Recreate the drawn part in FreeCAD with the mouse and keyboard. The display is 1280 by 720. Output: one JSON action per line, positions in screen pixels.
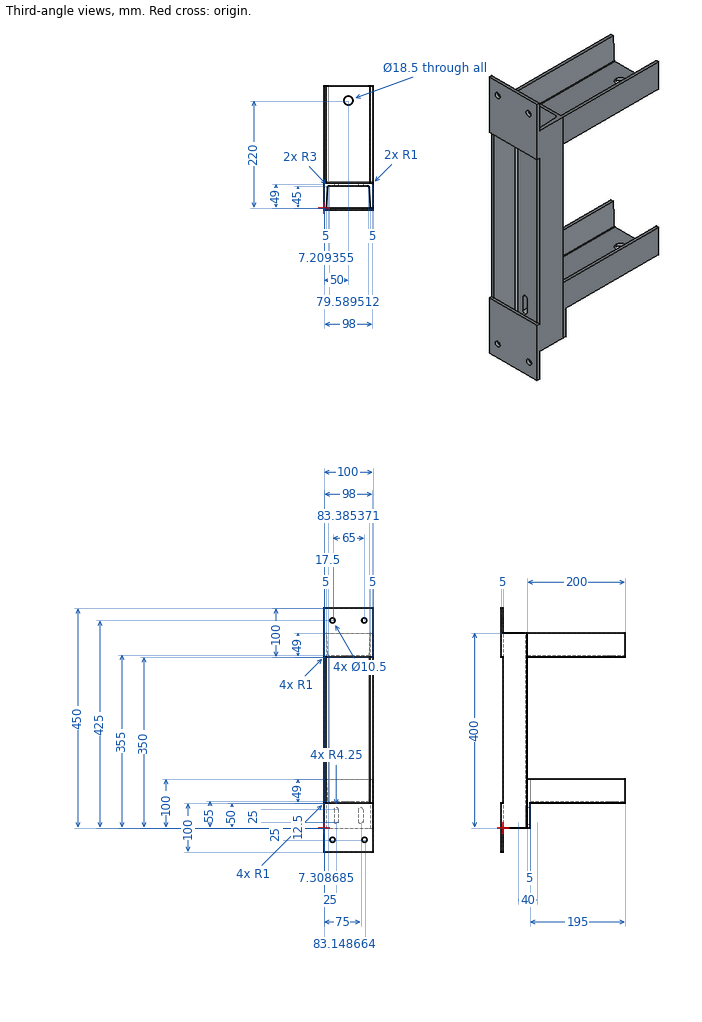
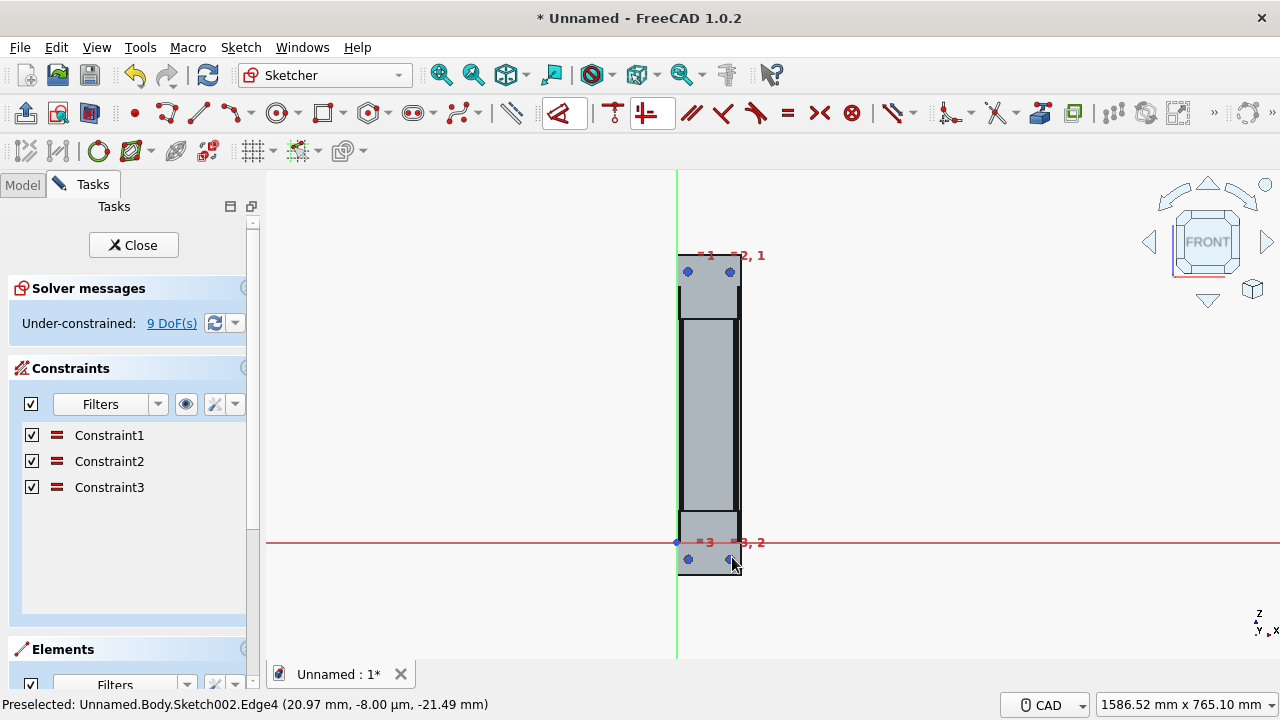
{"action": "left_click", "coordinate": [688, 272]}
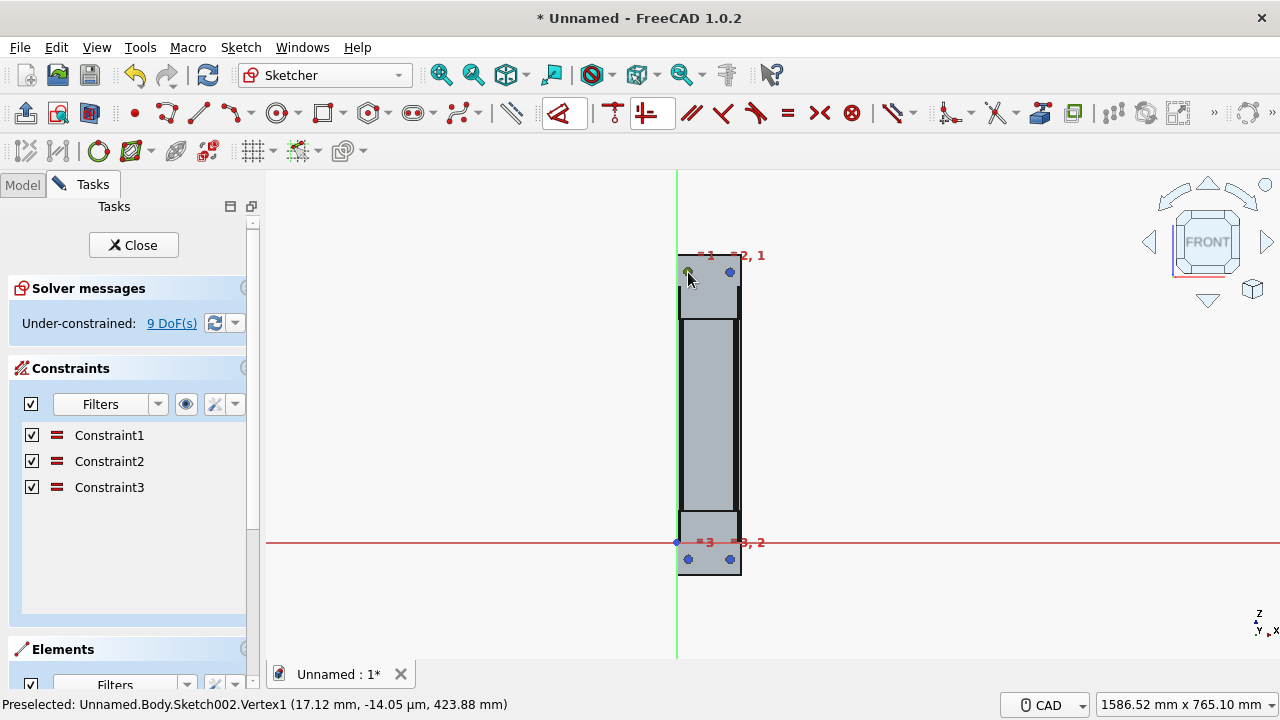
{"action": "left_click", "coordinate": [730, 272]}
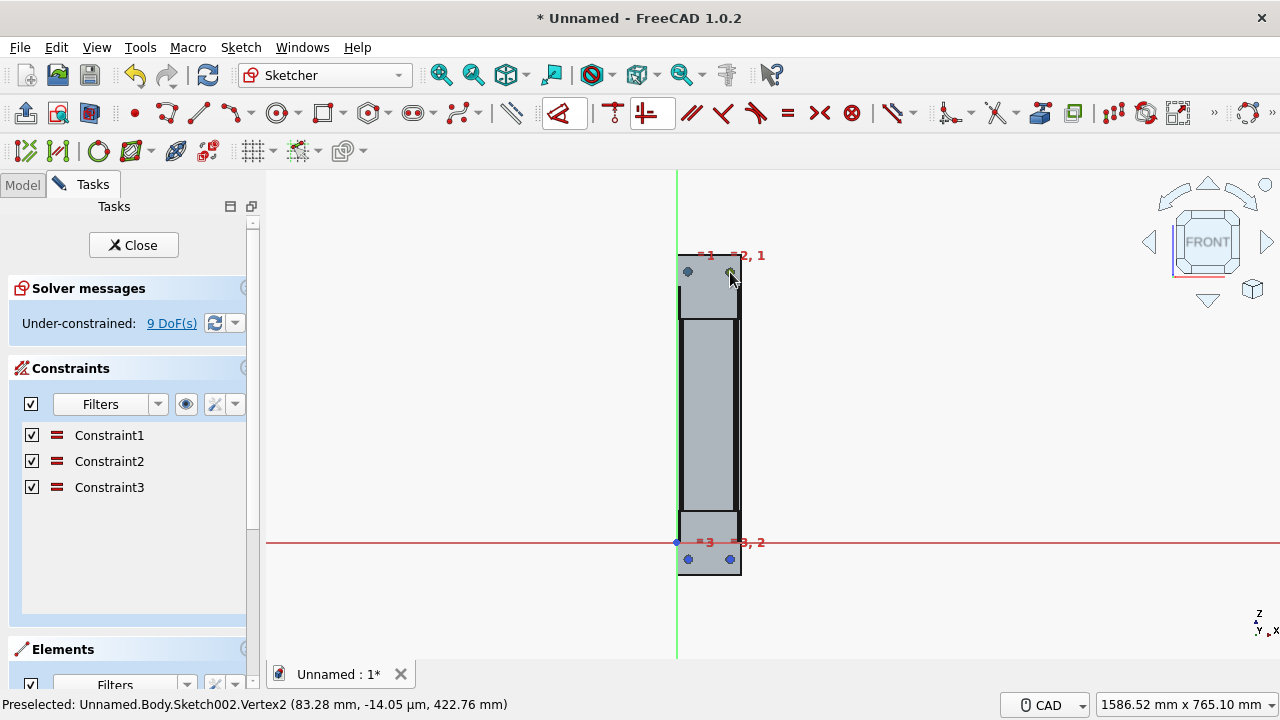
{"action": "key", "text": "h"}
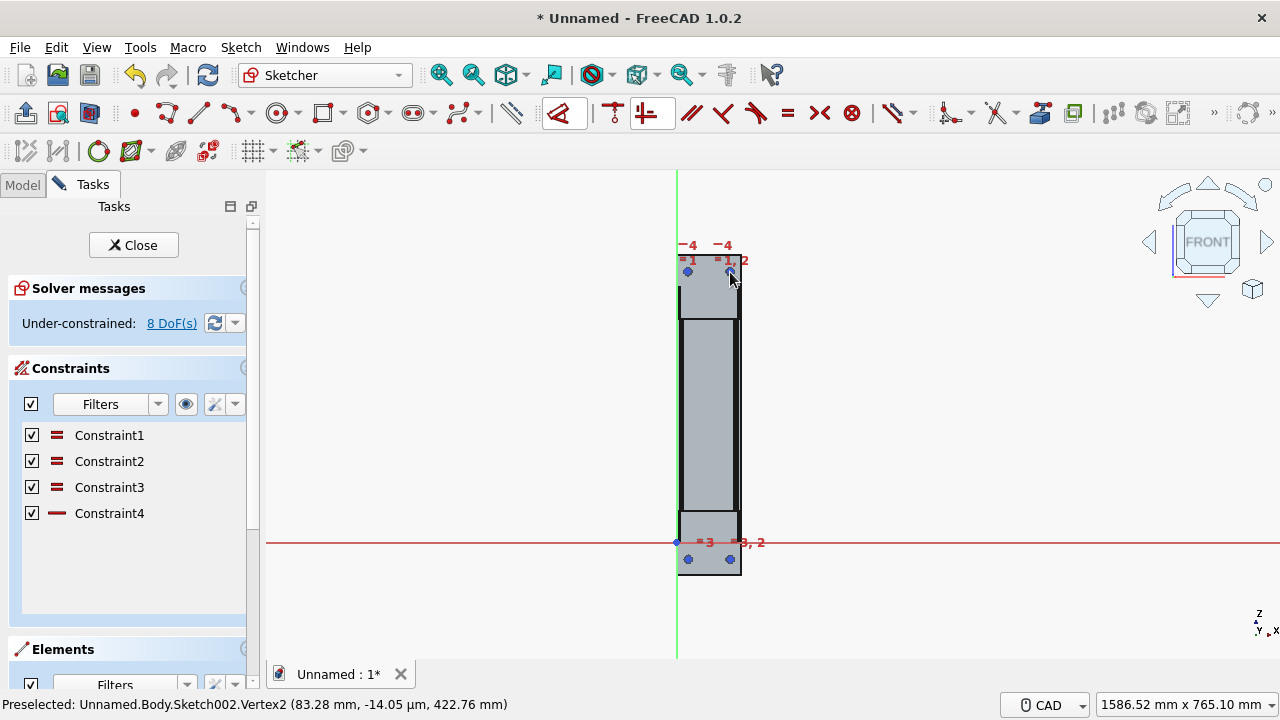
{"action": "left_click", "coordinate": [688, 272]}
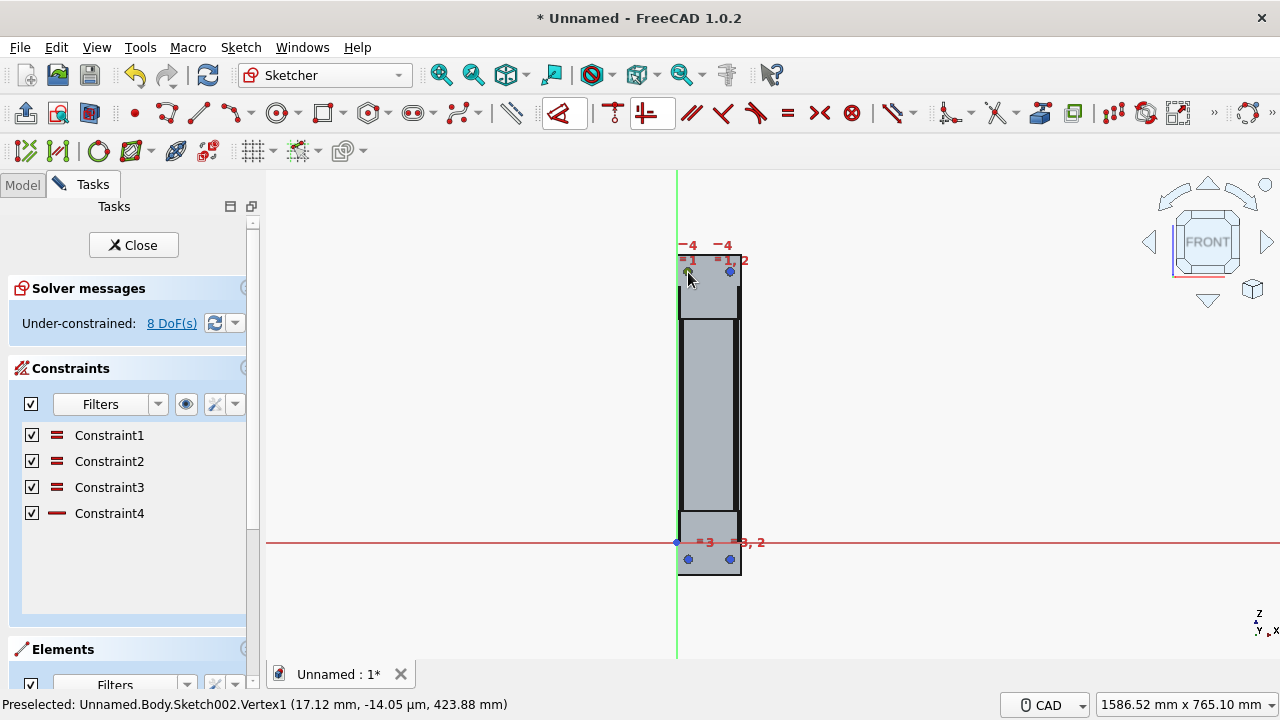
{"action": "left_click", "coordinate": [688, 559]}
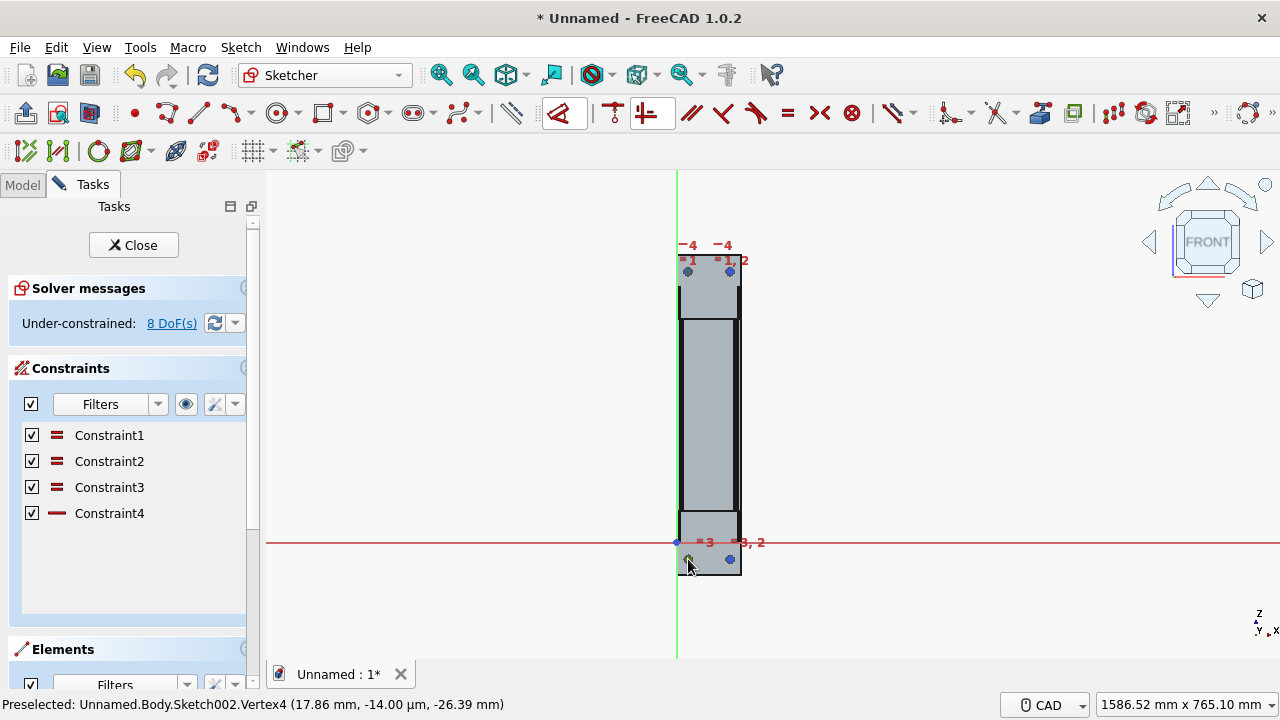
{"action": "left_click", "coordinate": [670, 114]}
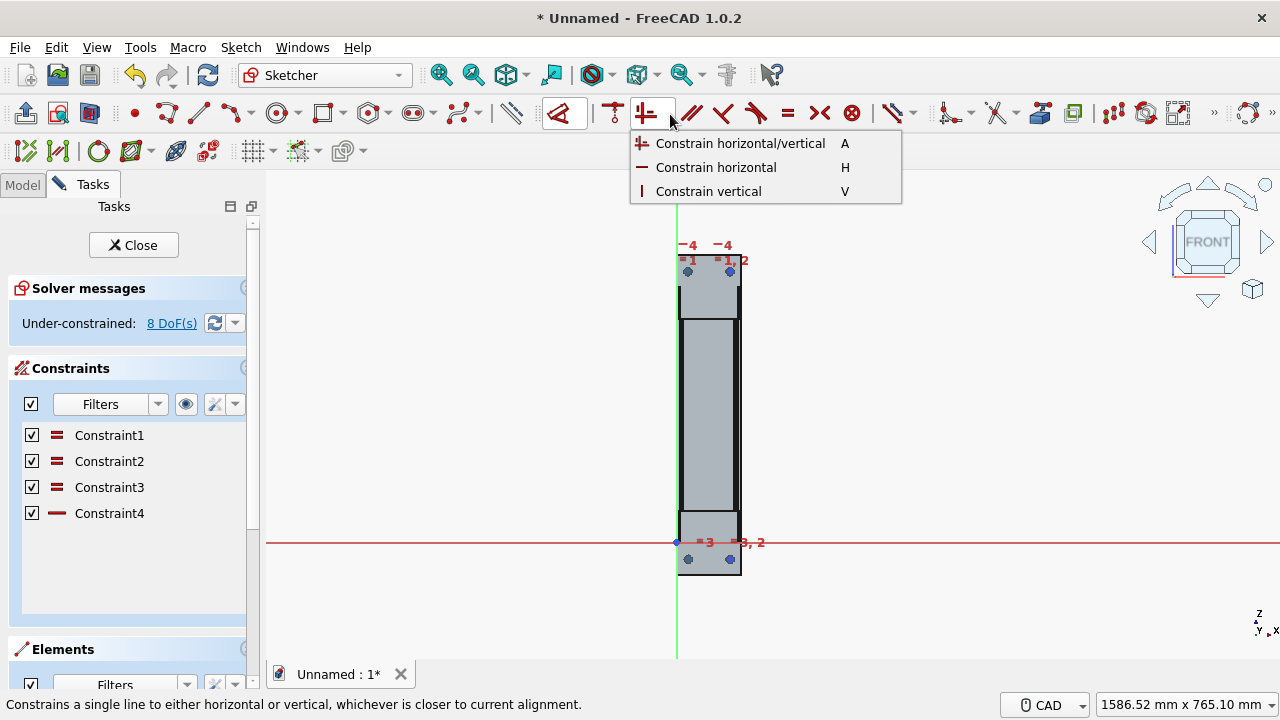
{"action": "left_click", "coordinate": [766, 191]}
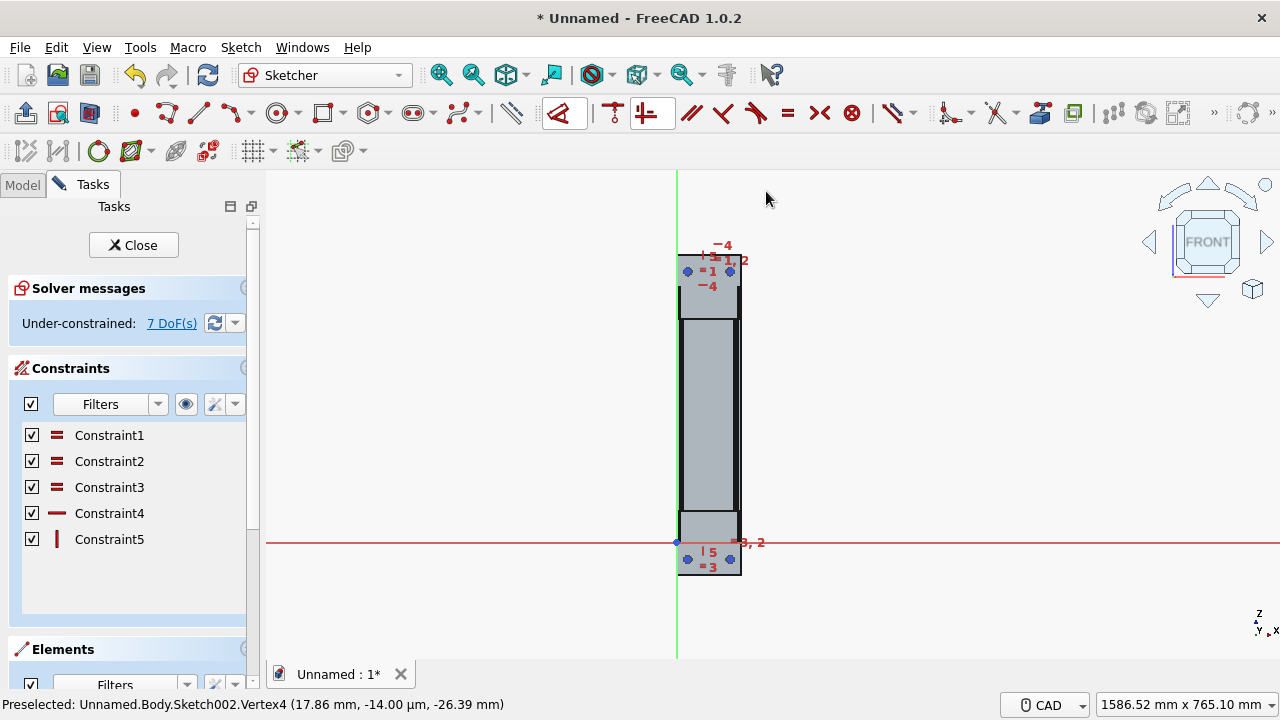
{"action": "left_click", "coordinate": [730, 560]}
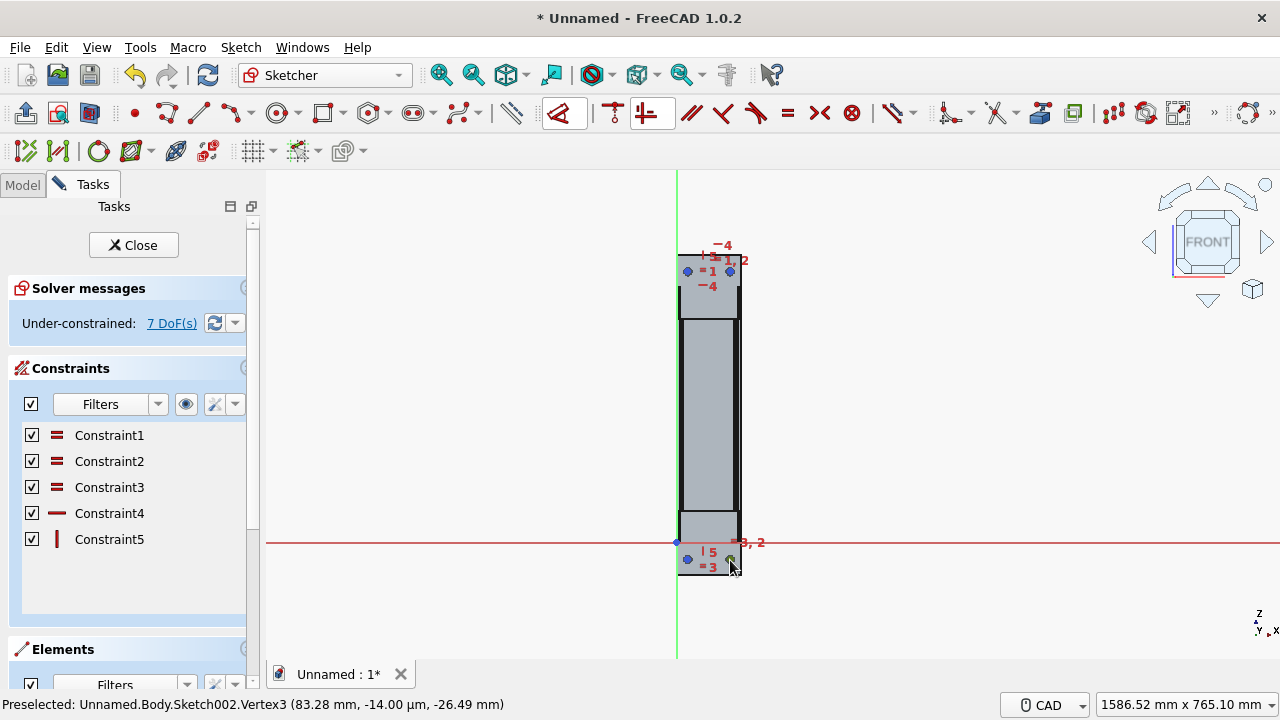
{"action": "left_click", "coordinate": [688, 559]}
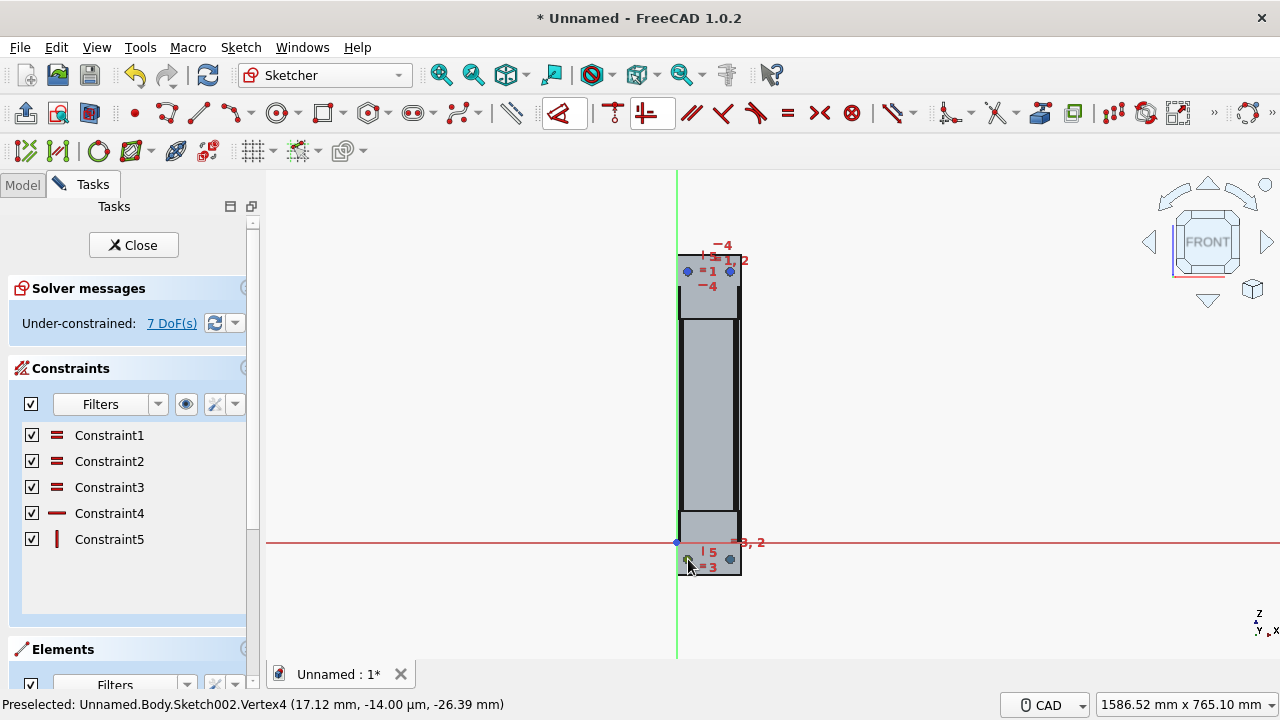
{"action": "key", "text": "h"}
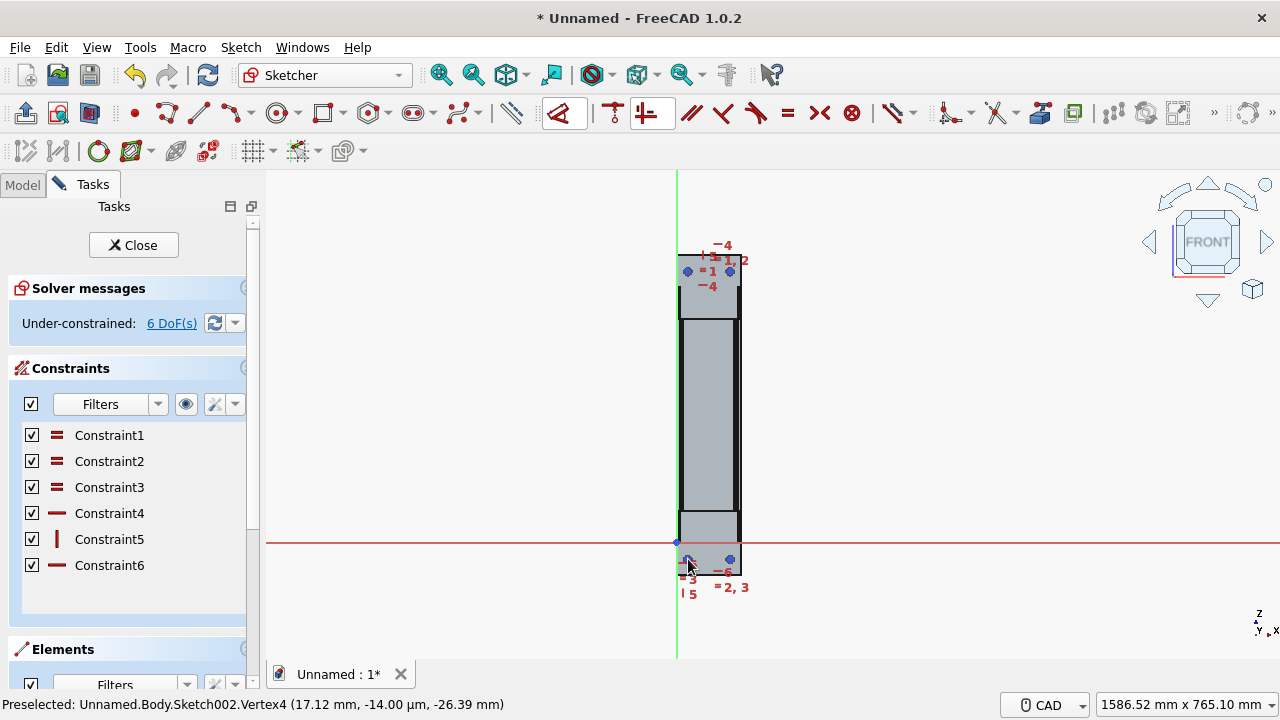
{"action": "scroll", "coordinate": [691, 274], "scroll_direction": "up", "scroll_amount": 9}